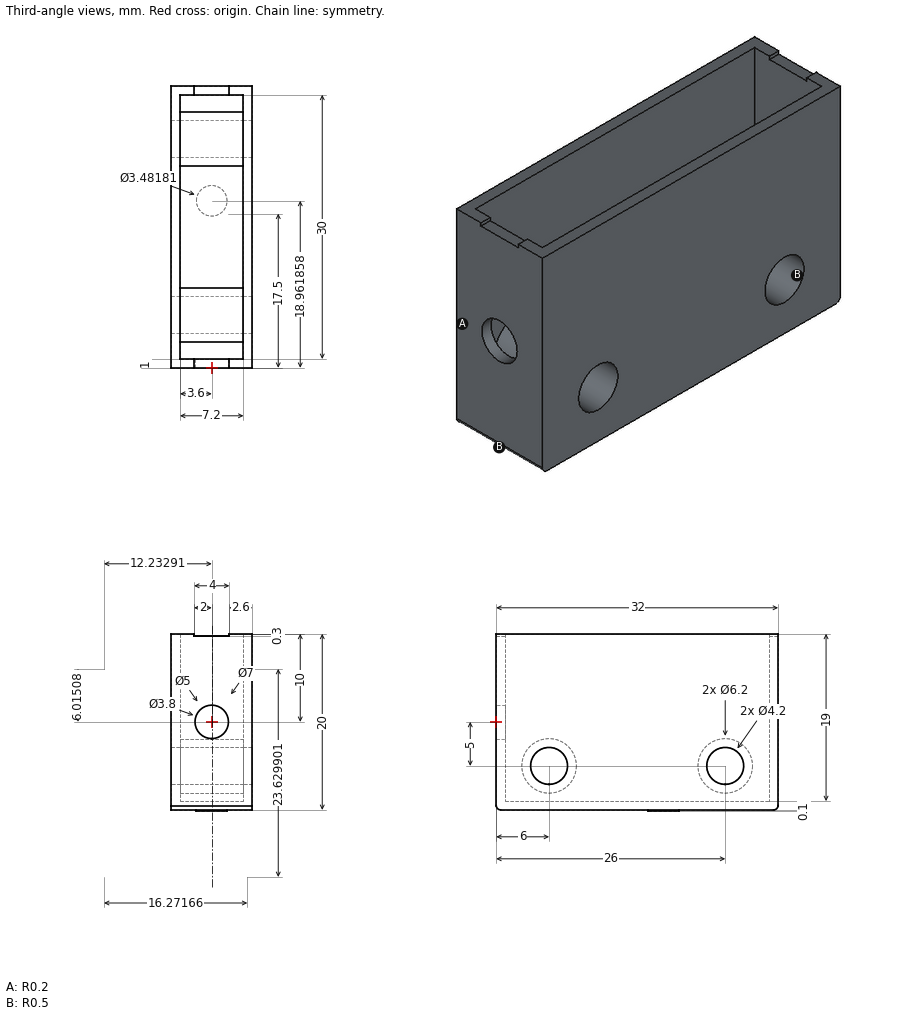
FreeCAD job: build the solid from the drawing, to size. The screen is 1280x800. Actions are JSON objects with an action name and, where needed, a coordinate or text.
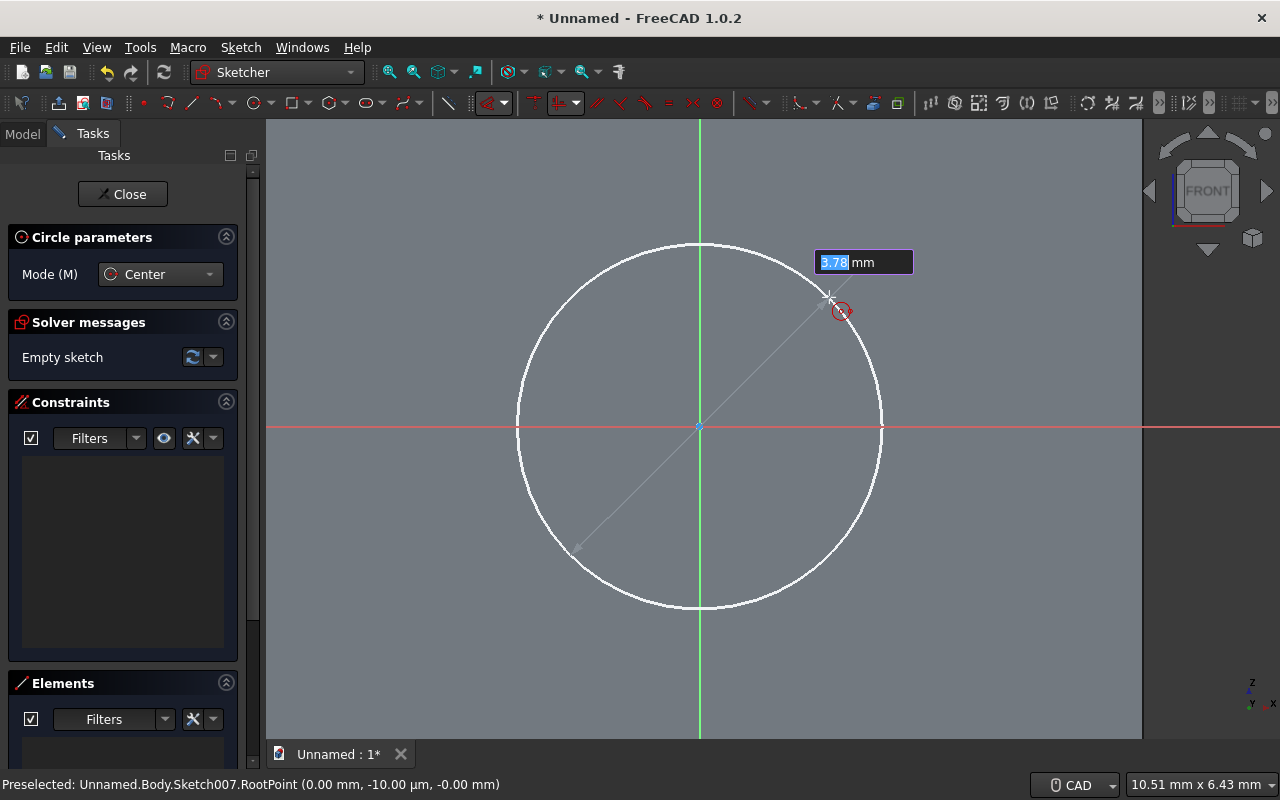
{"action": "type", "text": "3.8"}
{"action": "key", "text": "Return"}
{"action": "key", "text": "Escape"}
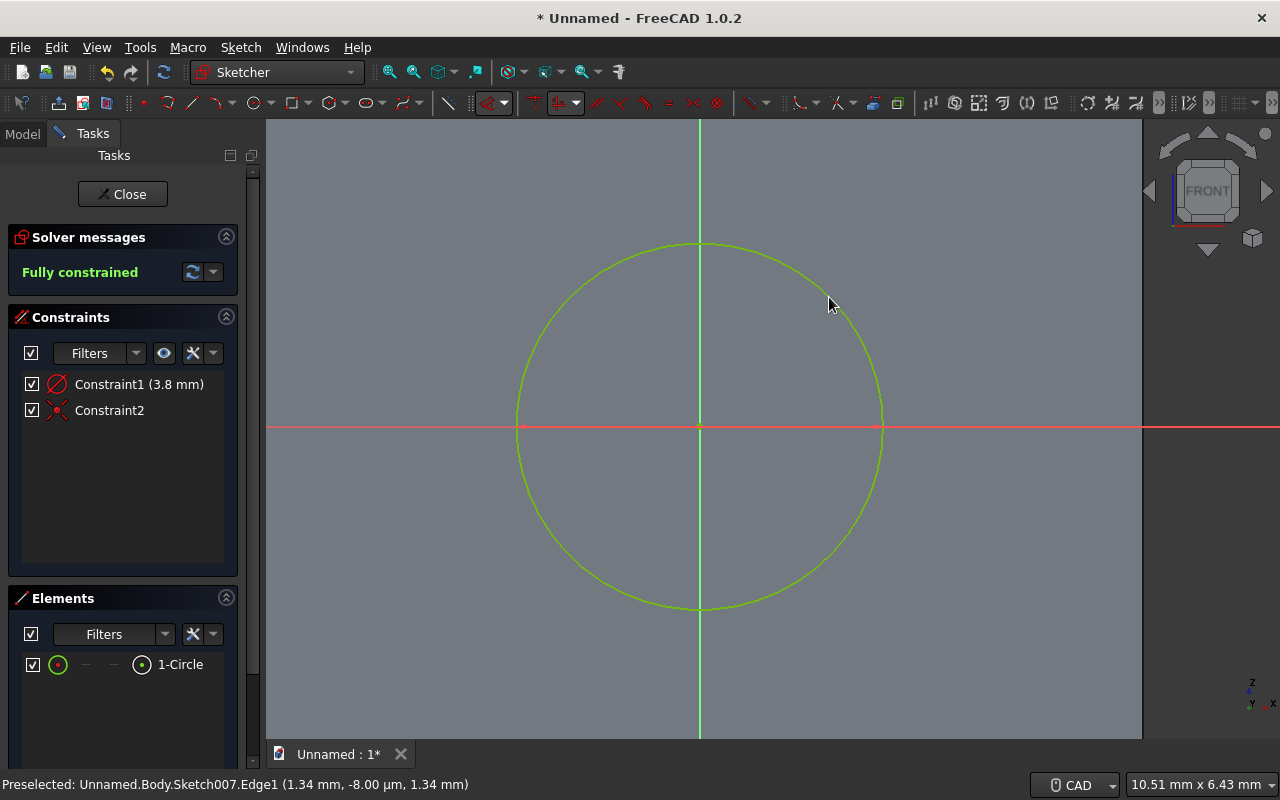
{"action": "left_click", "coordinate": [123, 194]}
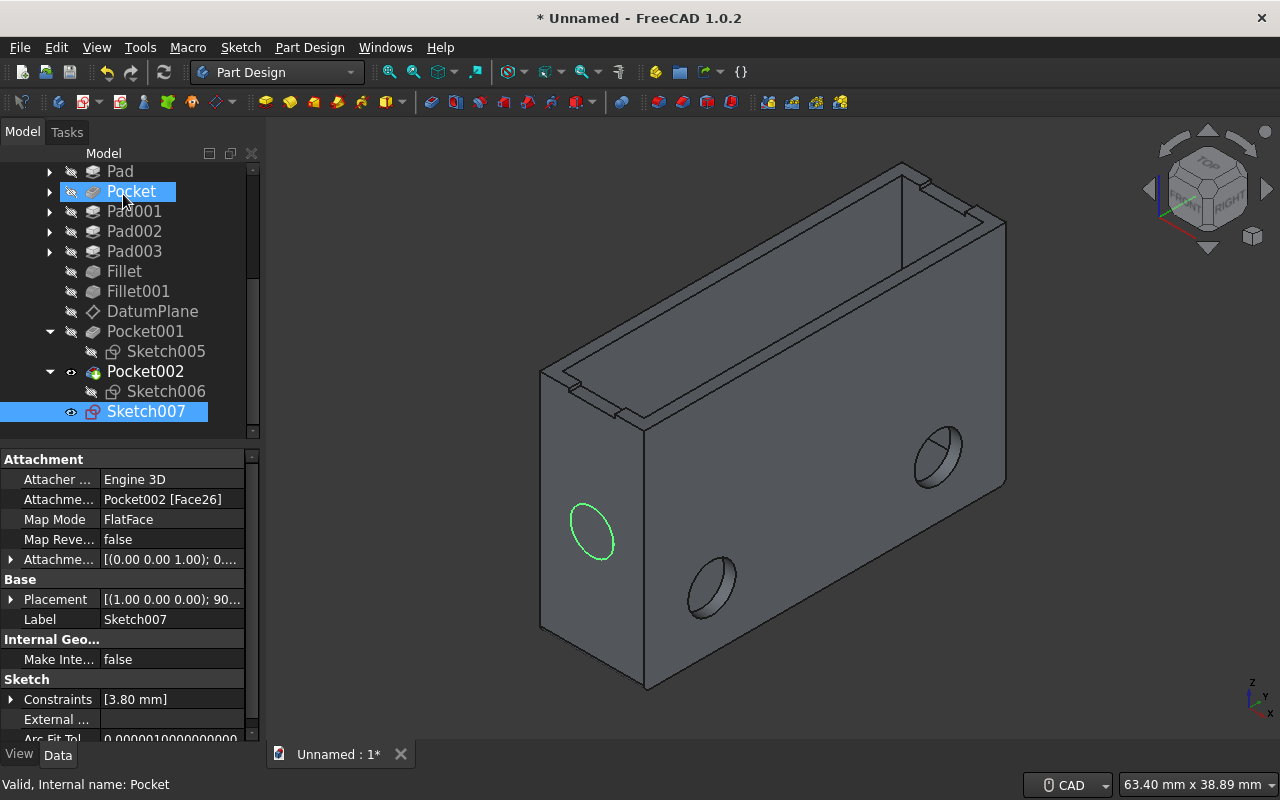
{"action": "left_click", "coordinate": [432, 102]}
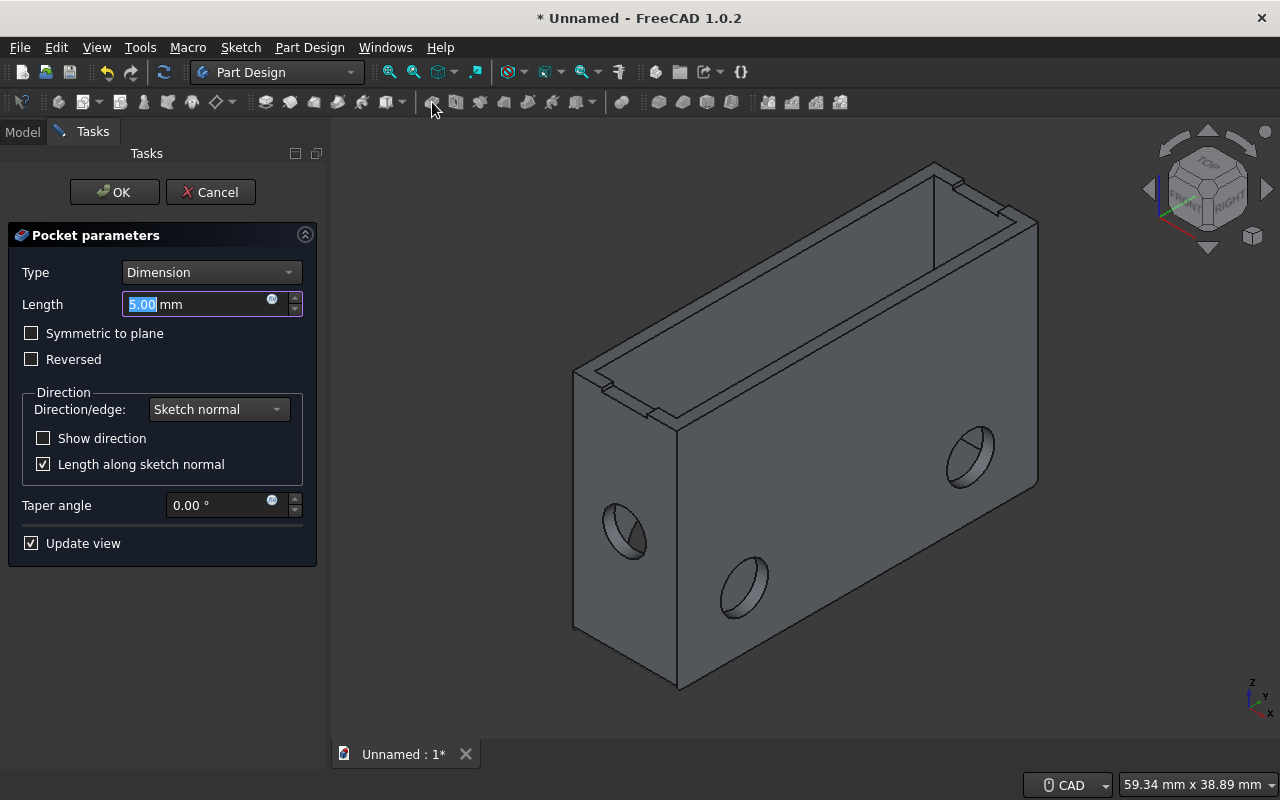
{"action": "type", "text": "17.5"}
{"action": "key", "text": "Tab"}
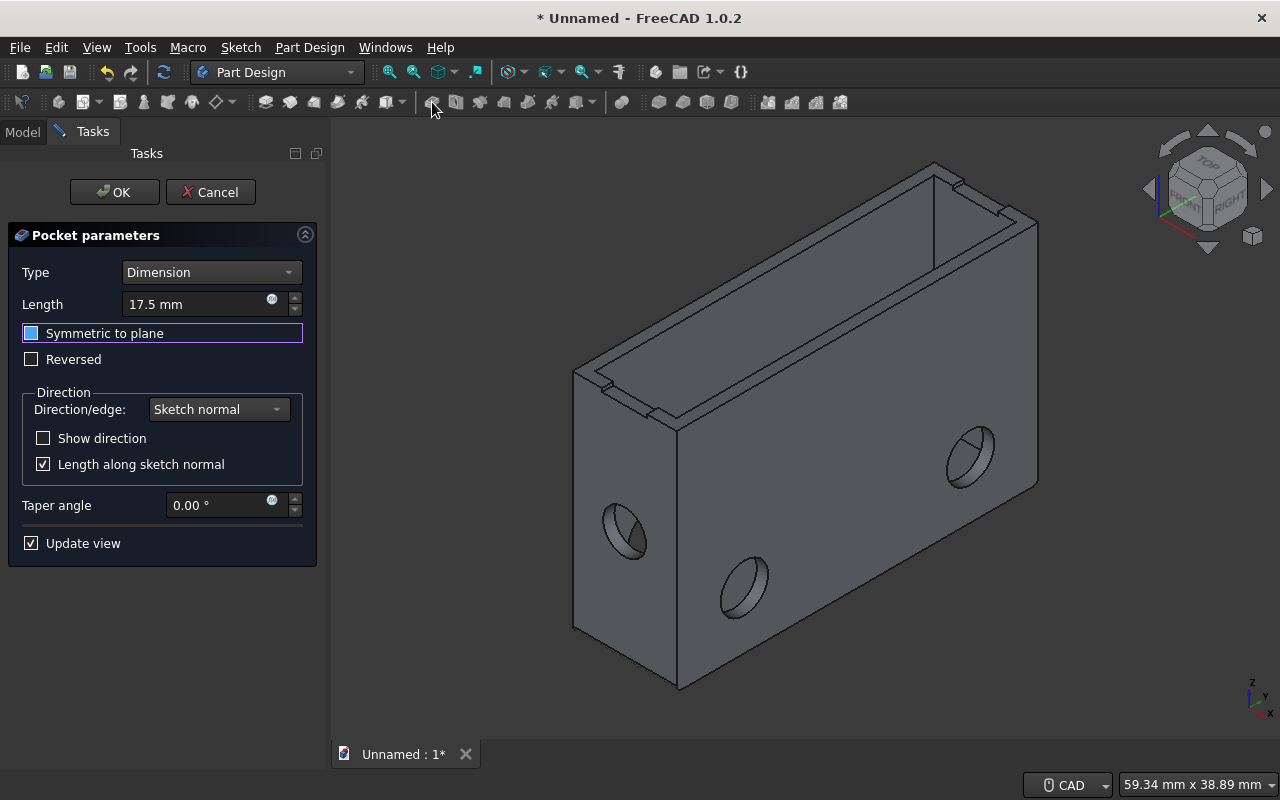
{"action": "left_click", "coordinate": [115, 192]}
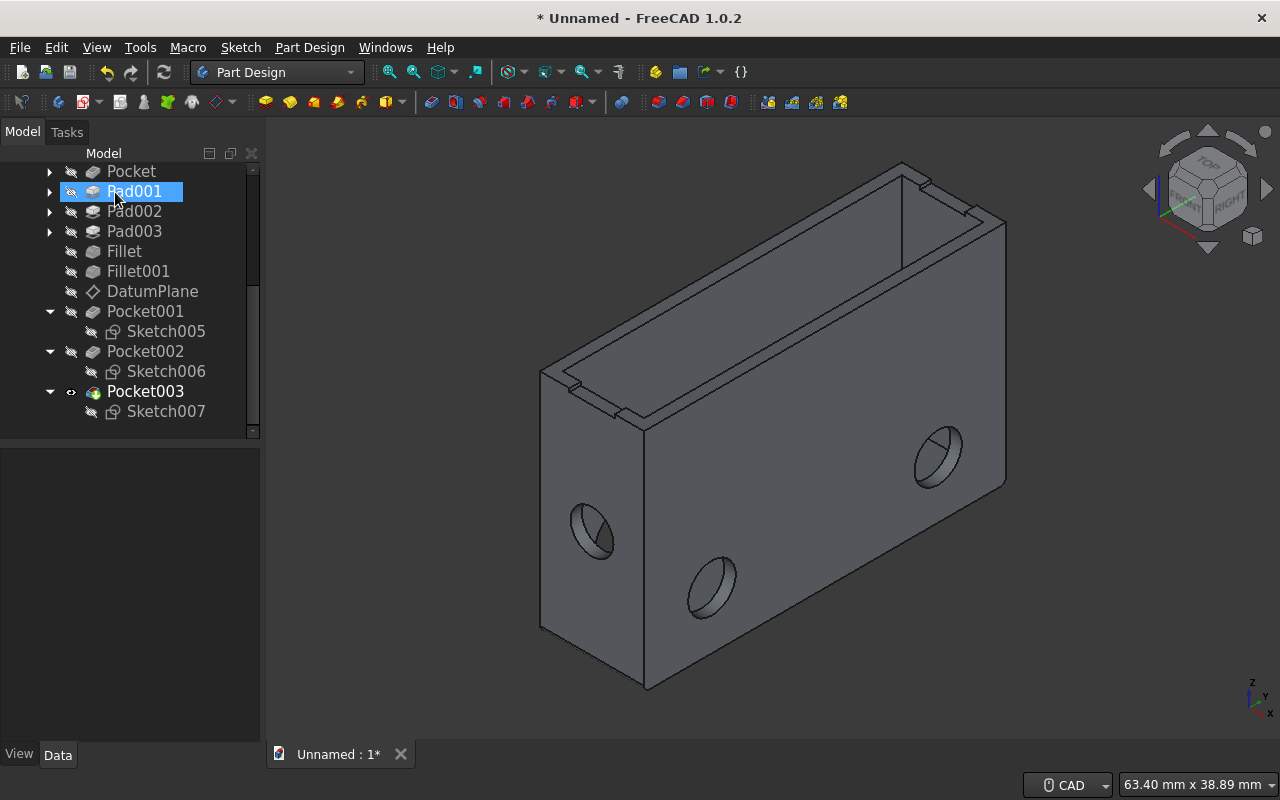
{"action": "scroll", "coordinate": [140, 287], "scroll_direction": "down", "scroll_amount": 3}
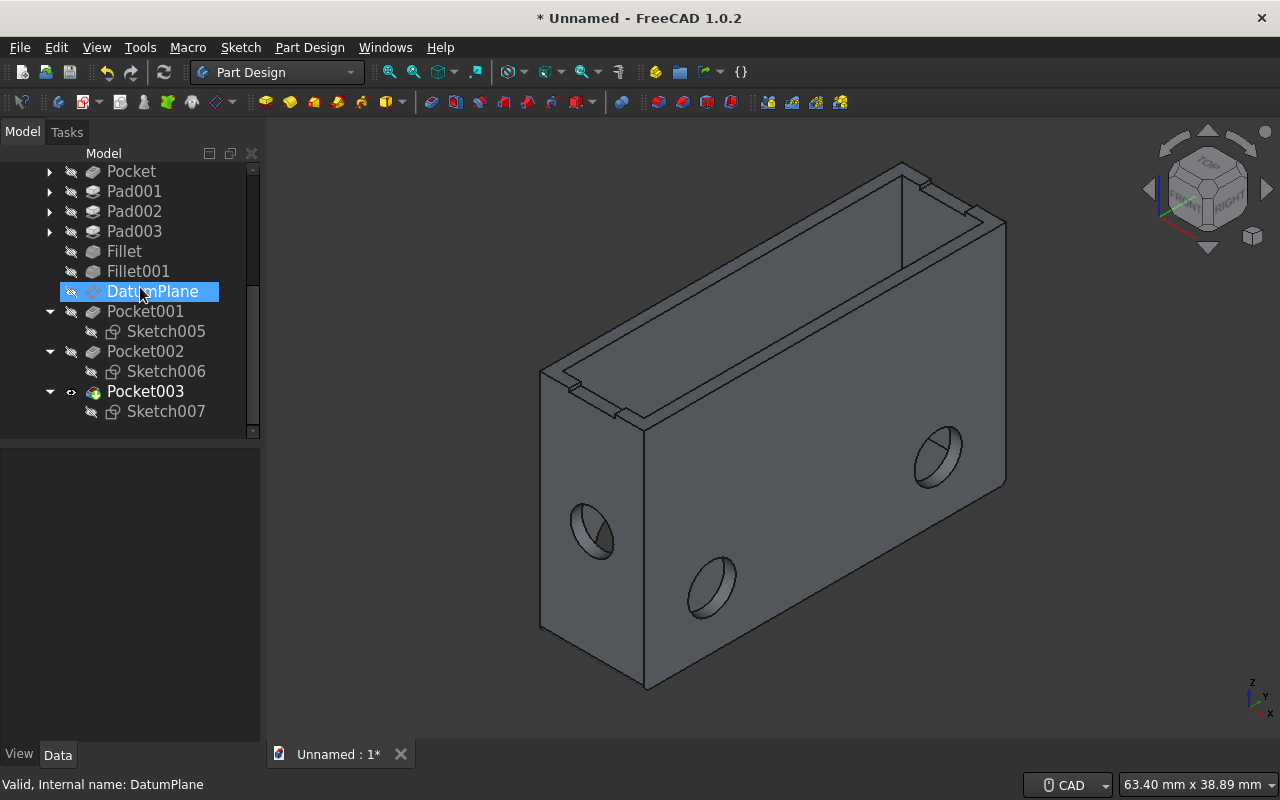
{"action": "scroll", "coordinate": [140, 287], "scroll_direction": "up", "scroll_amount": 15}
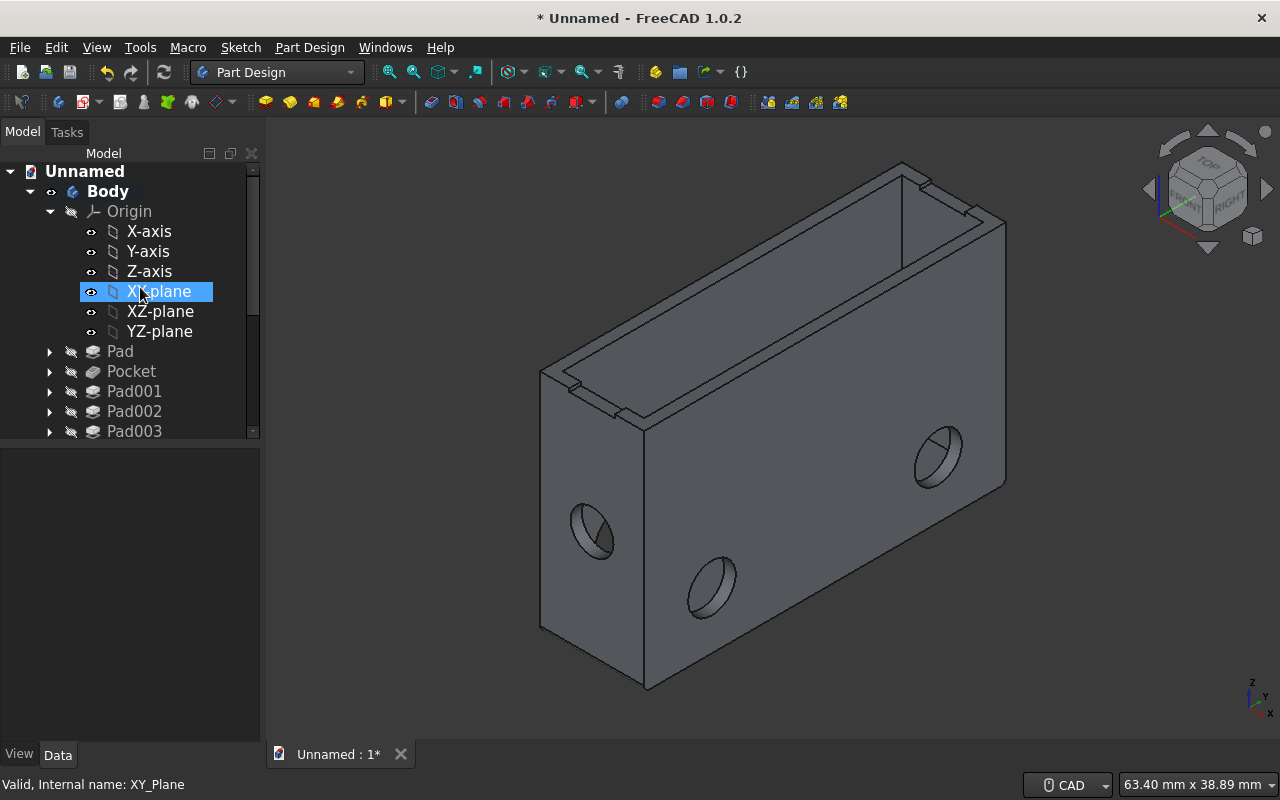
{"action": "left_click", "coordinate": [136, 332]}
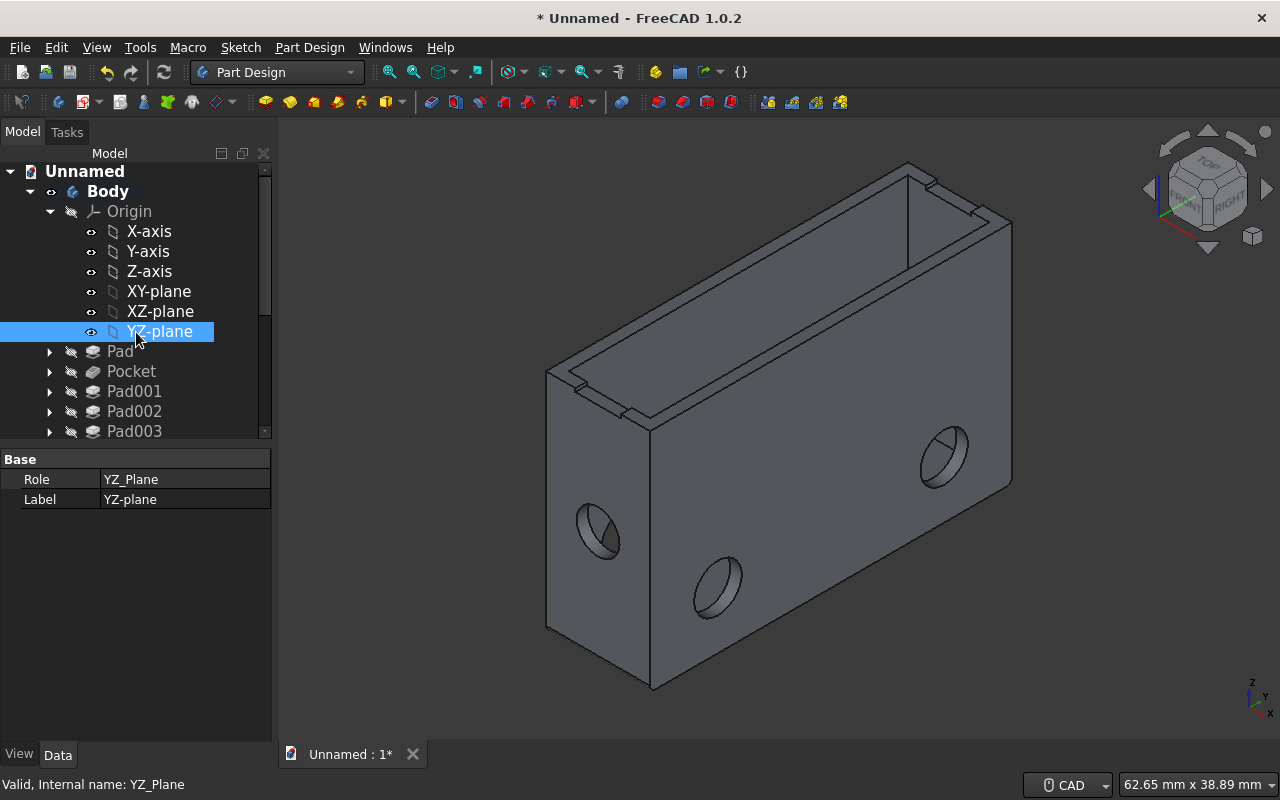
{"action": "left_click", "coordinate": [216, 102]}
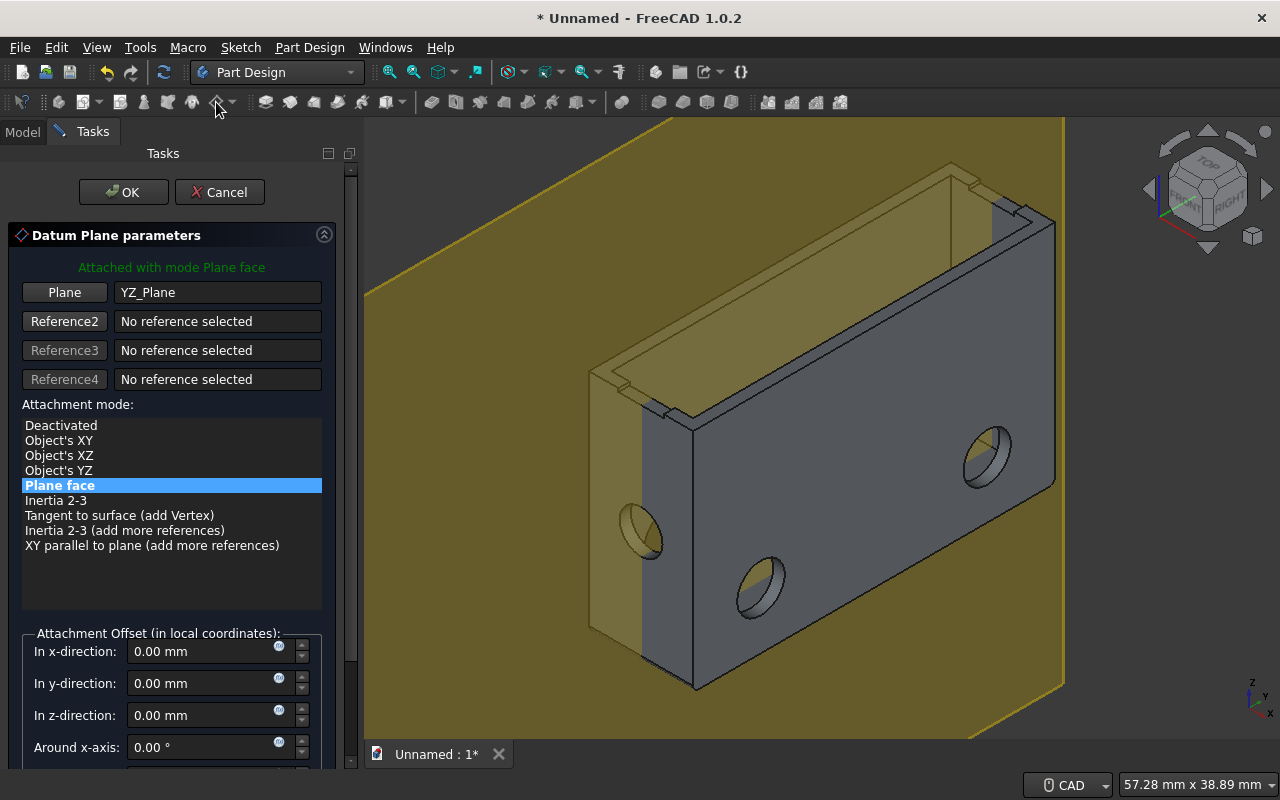
{"action": "triple_click", "coordinate": [210, 715]}